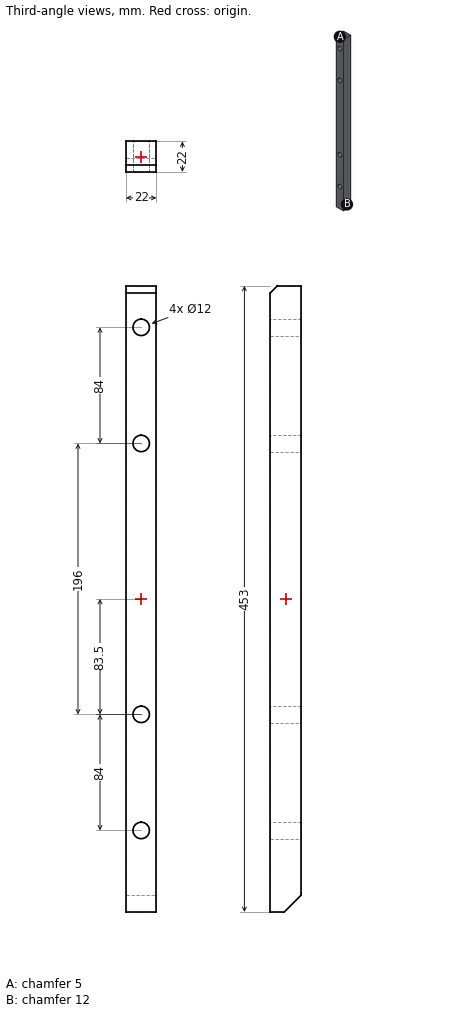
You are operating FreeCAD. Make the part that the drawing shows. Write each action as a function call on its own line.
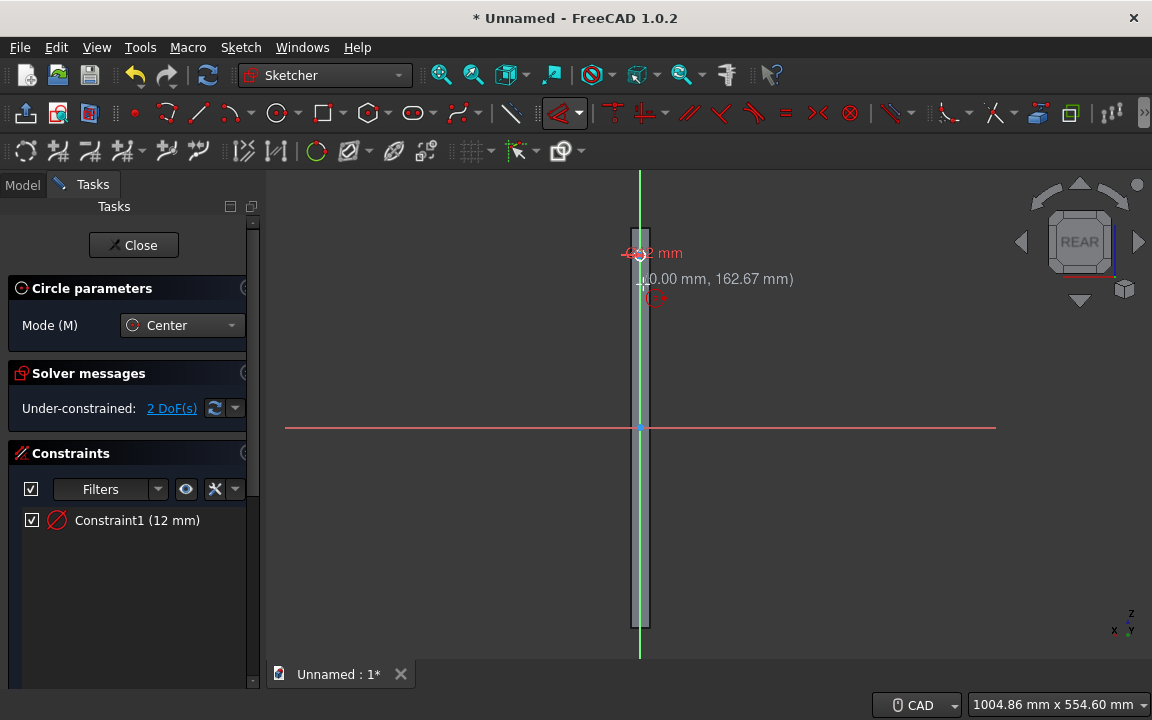
click(640, 329)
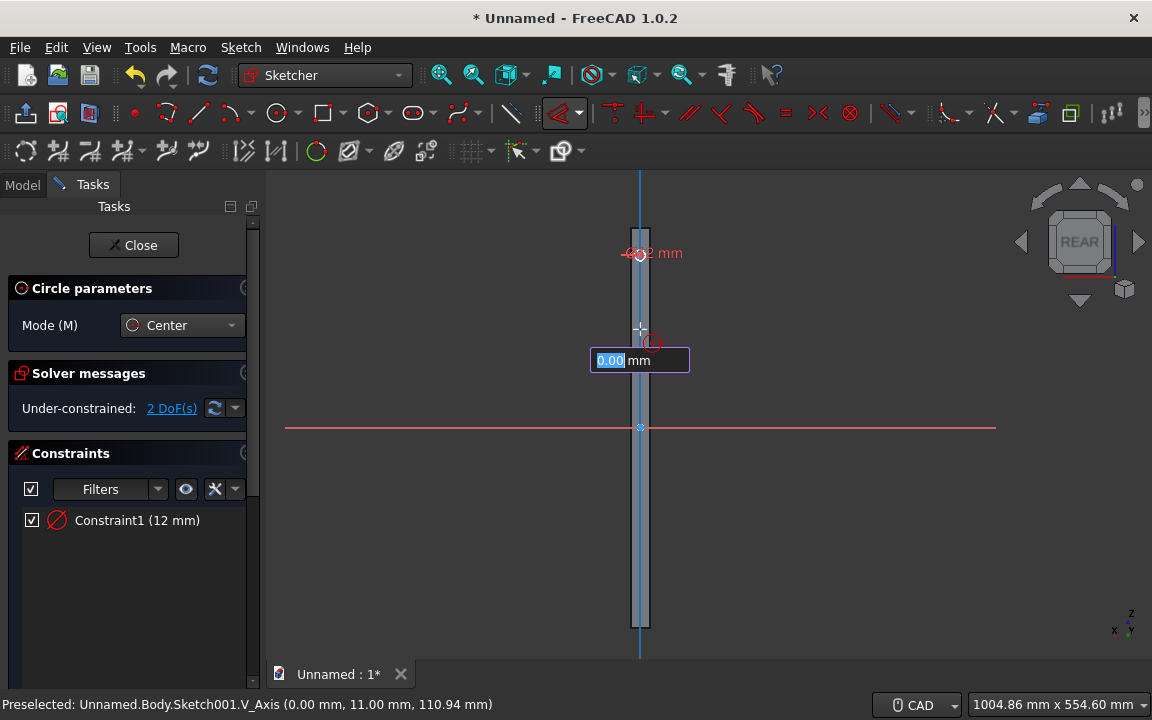
scroll(645, 327, up, 6)
move(646, 326)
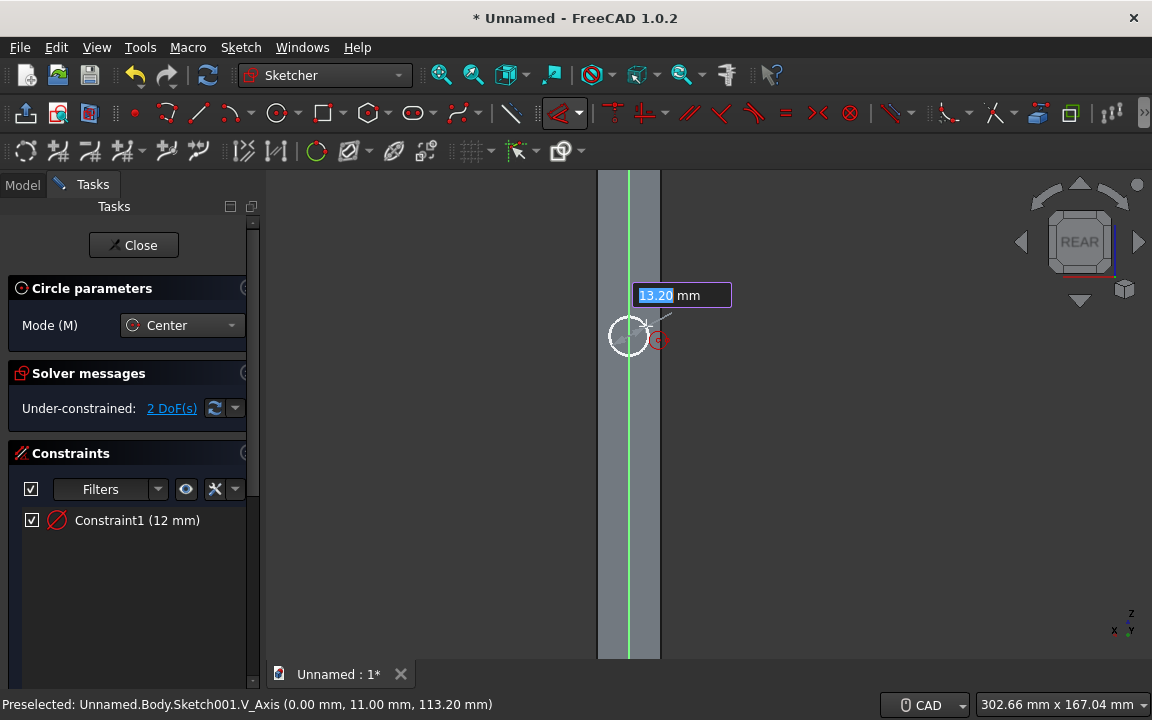
text(12)
key(Return)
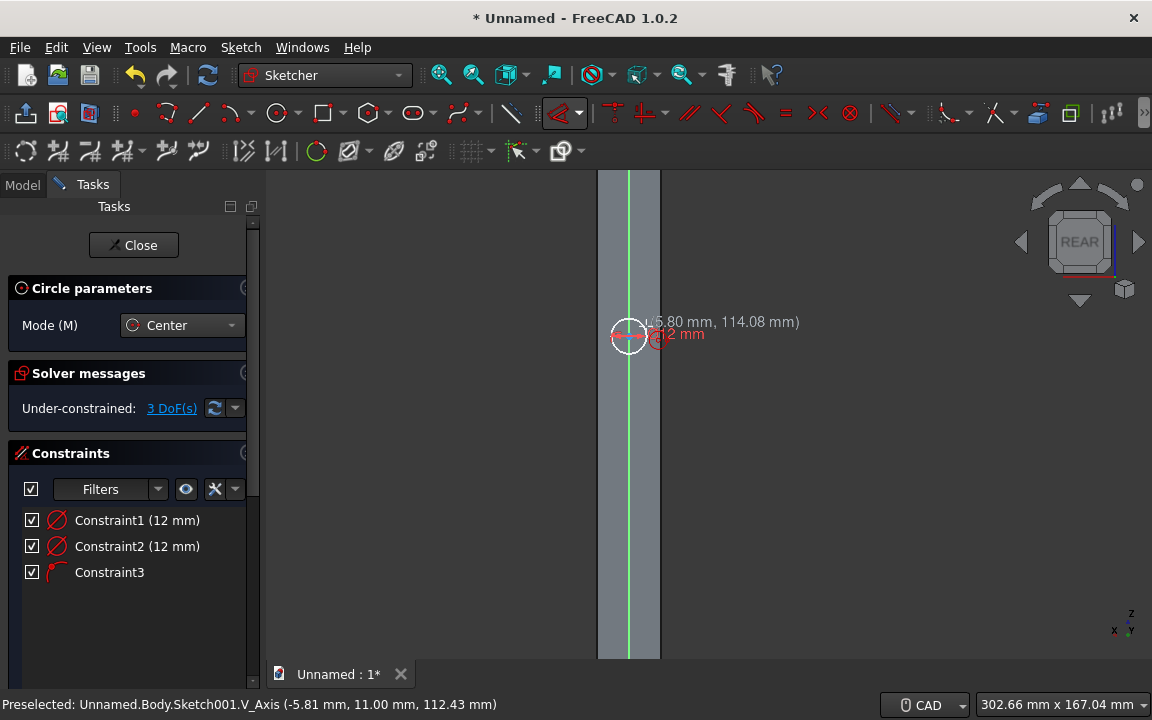
scroll(645, 327, down, 6)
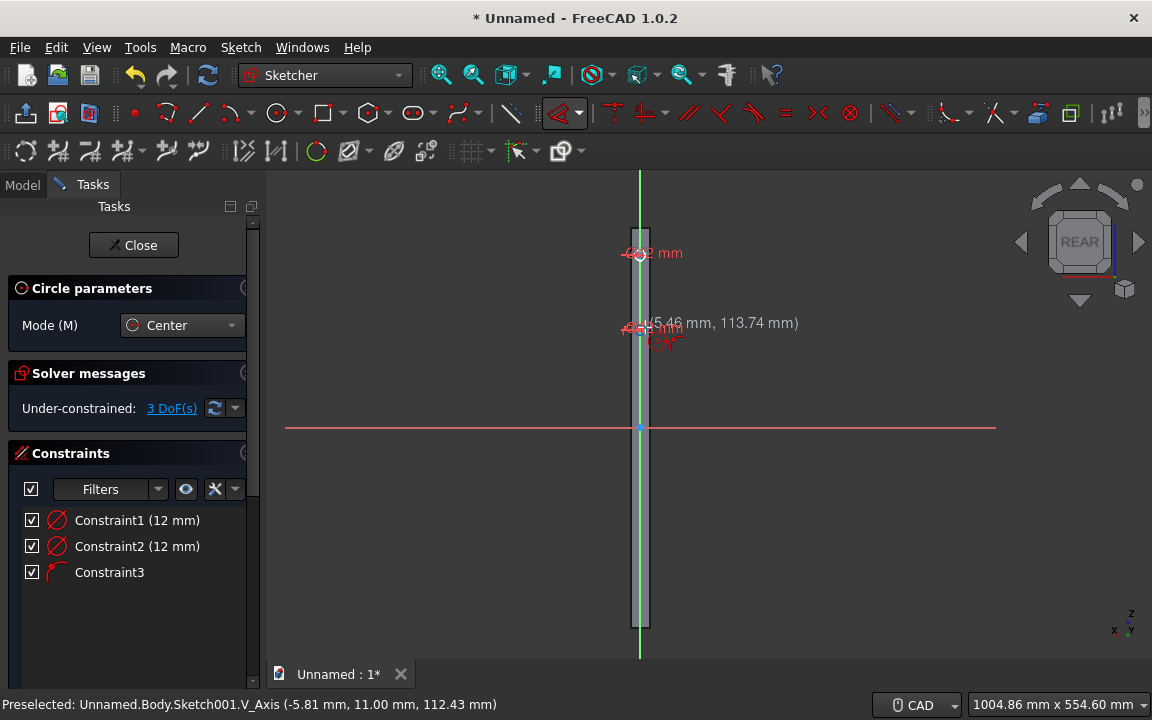
scroll(640, 501, up, 8)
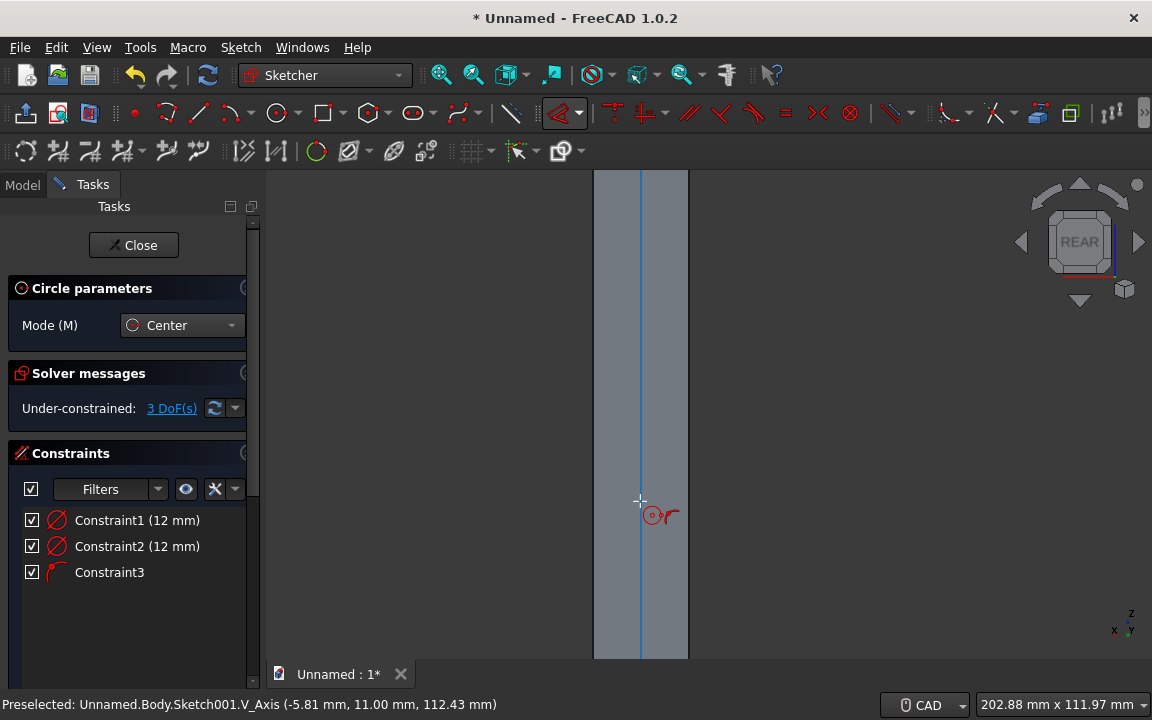
scroll(640, 501, down, 8)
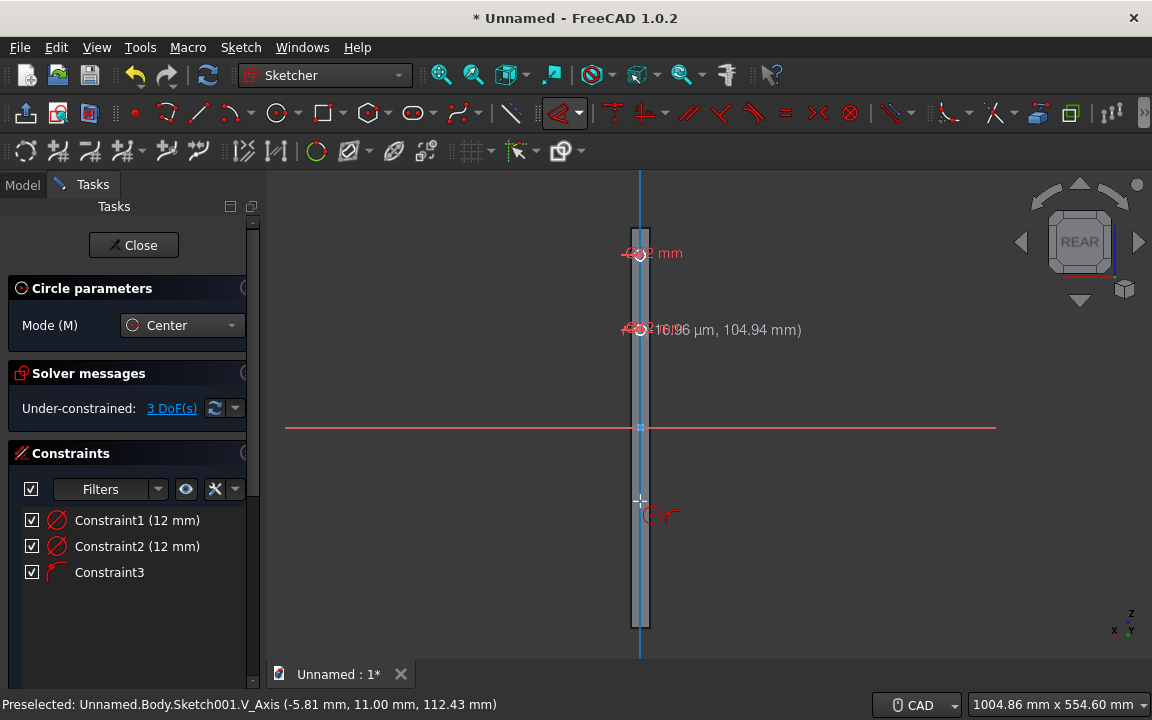
click(640, 501)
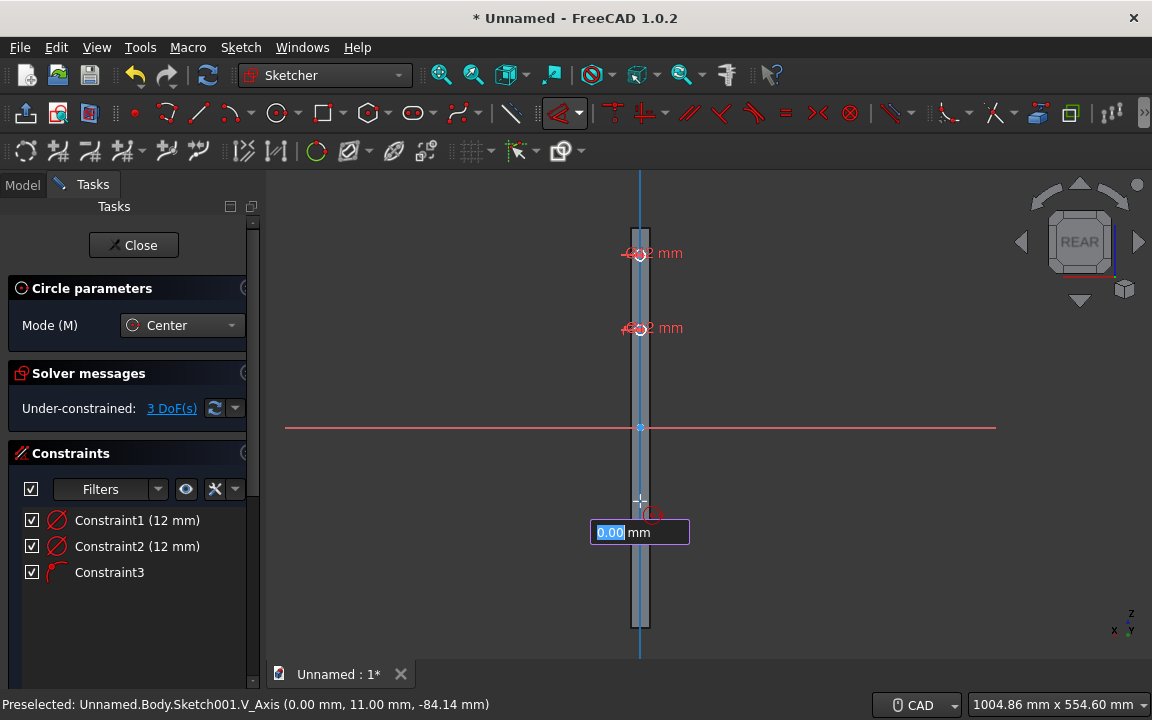
scroll(645, 500, up, 6)
move(646, 497)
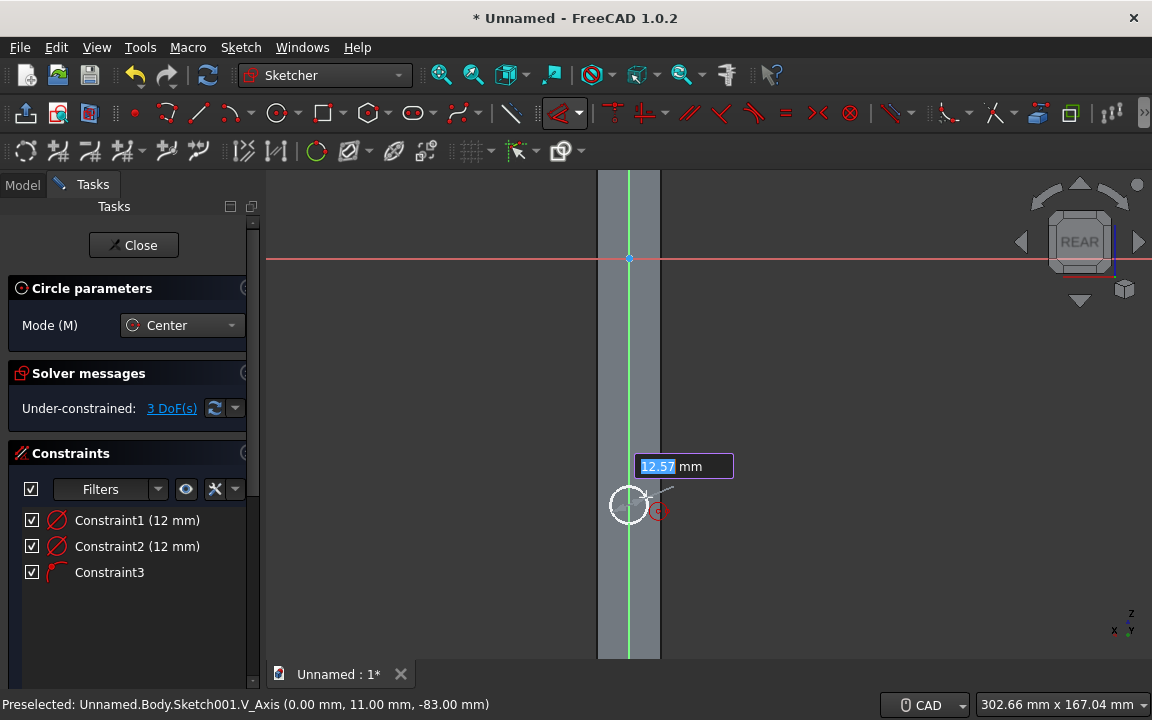
text(12)
key(Return)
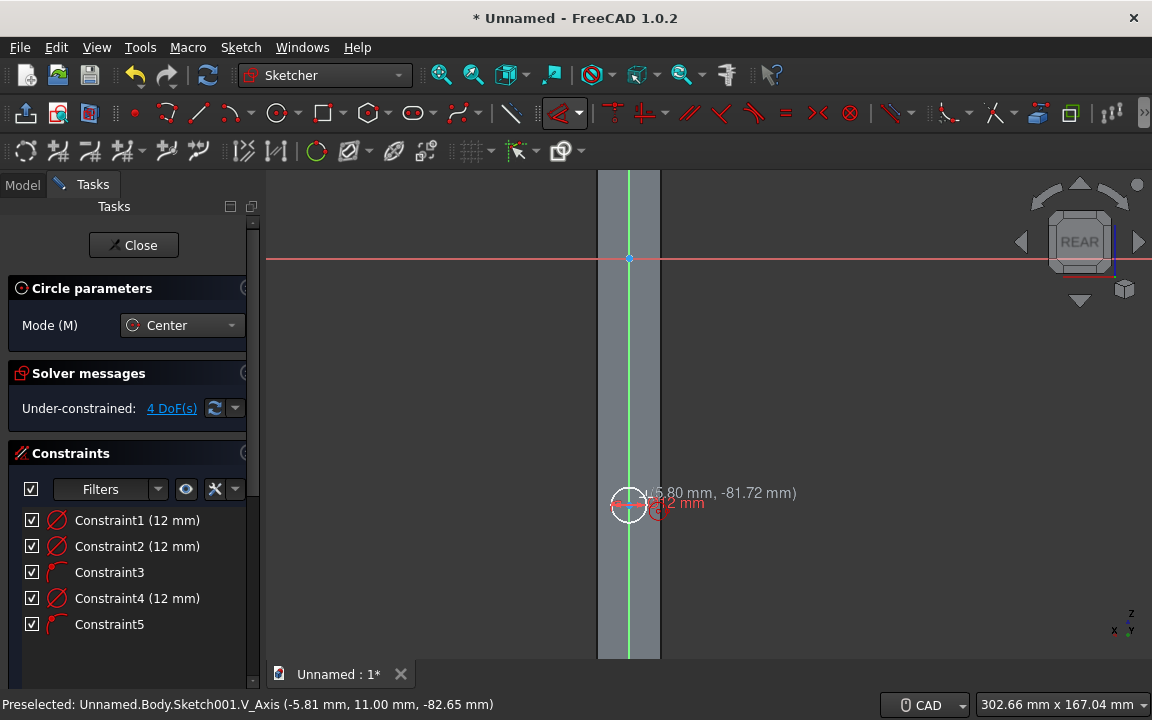
scroll(645, 500, down, 6)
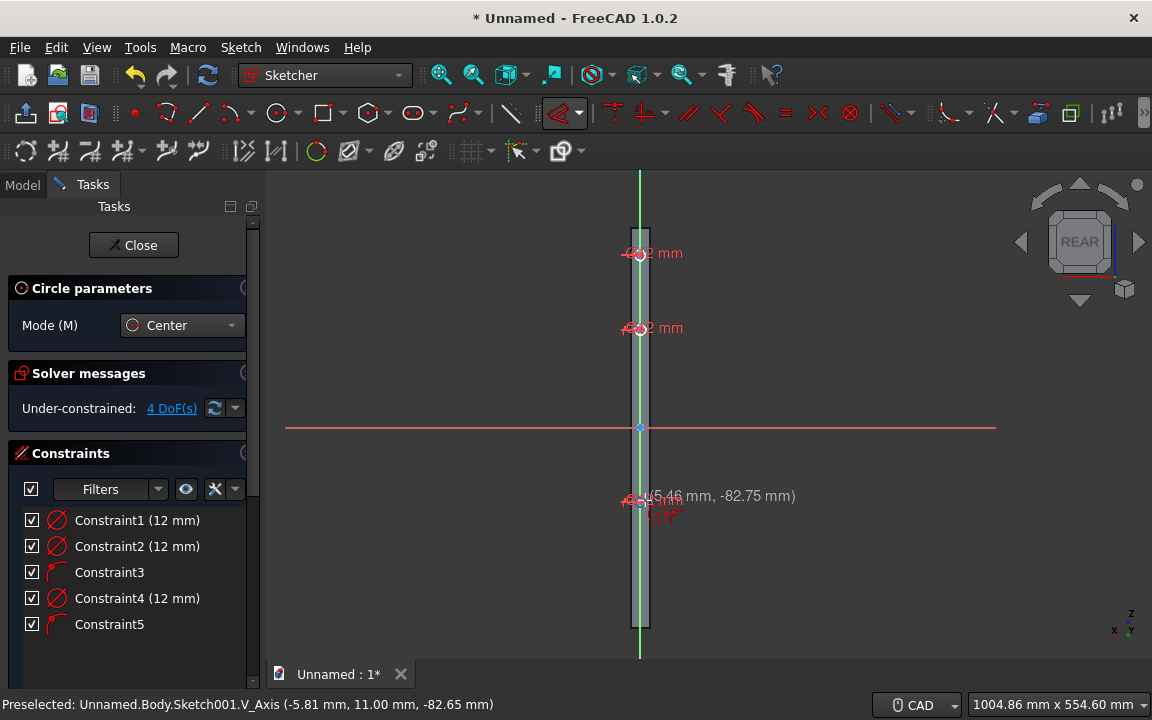
scroll(640, 576, up, 8)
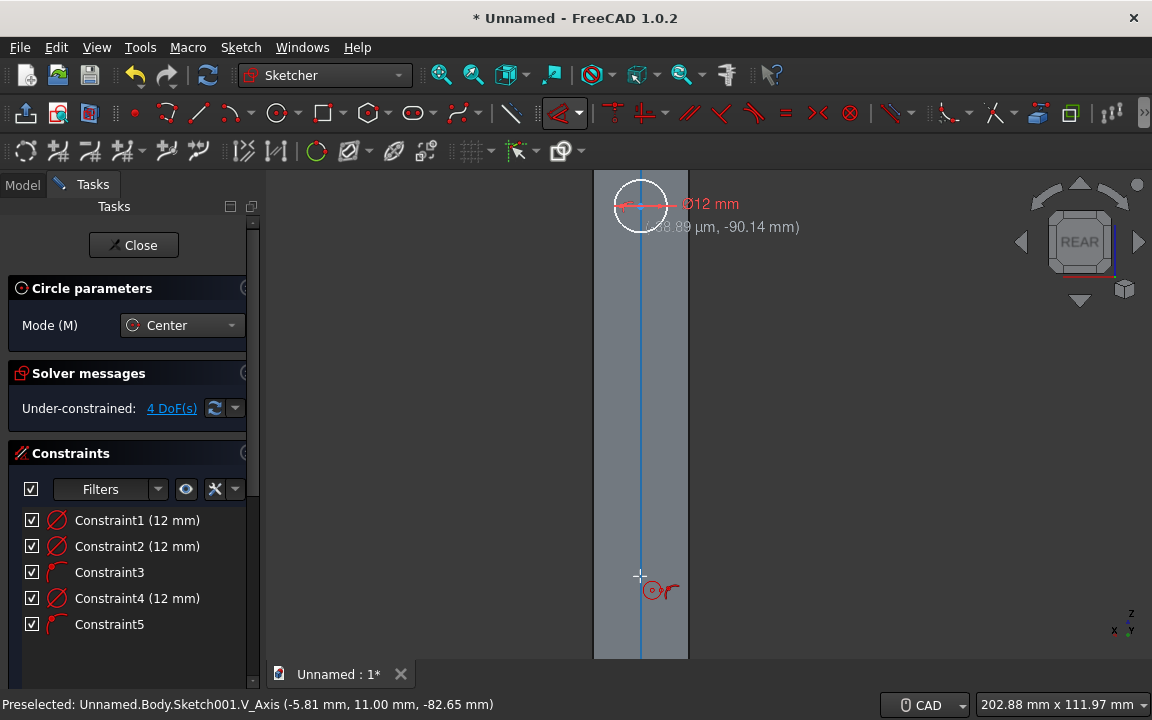
scroll(640, 576, down, 8)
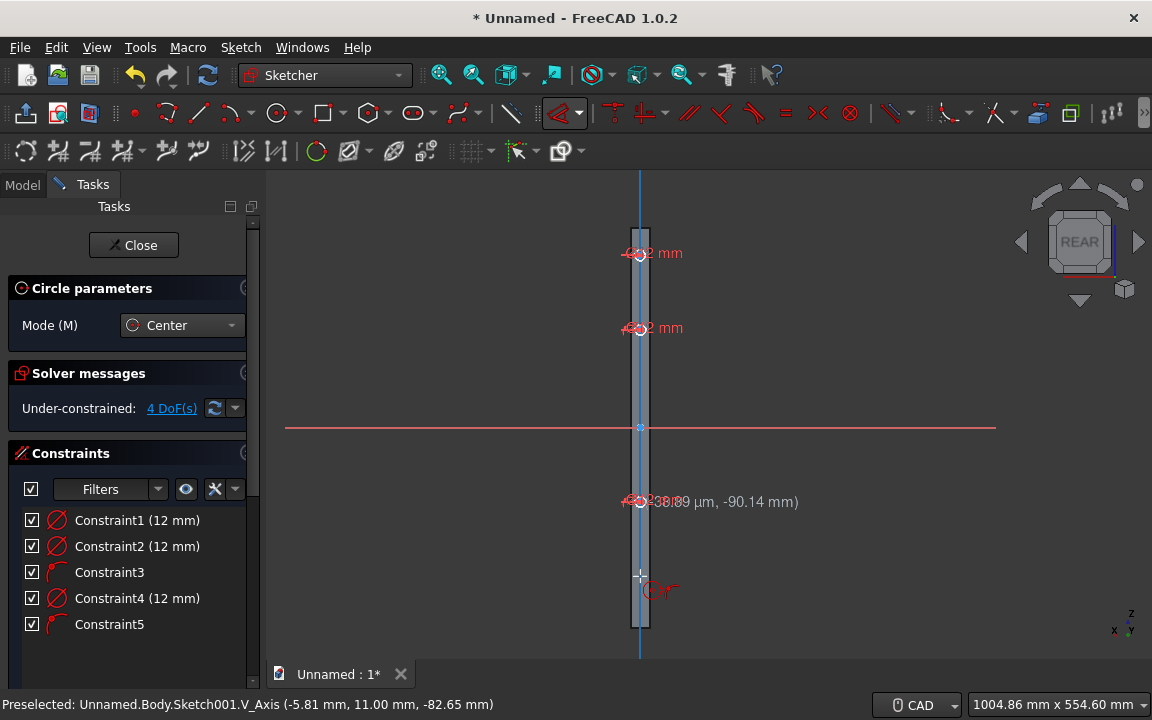
click(640, 576)